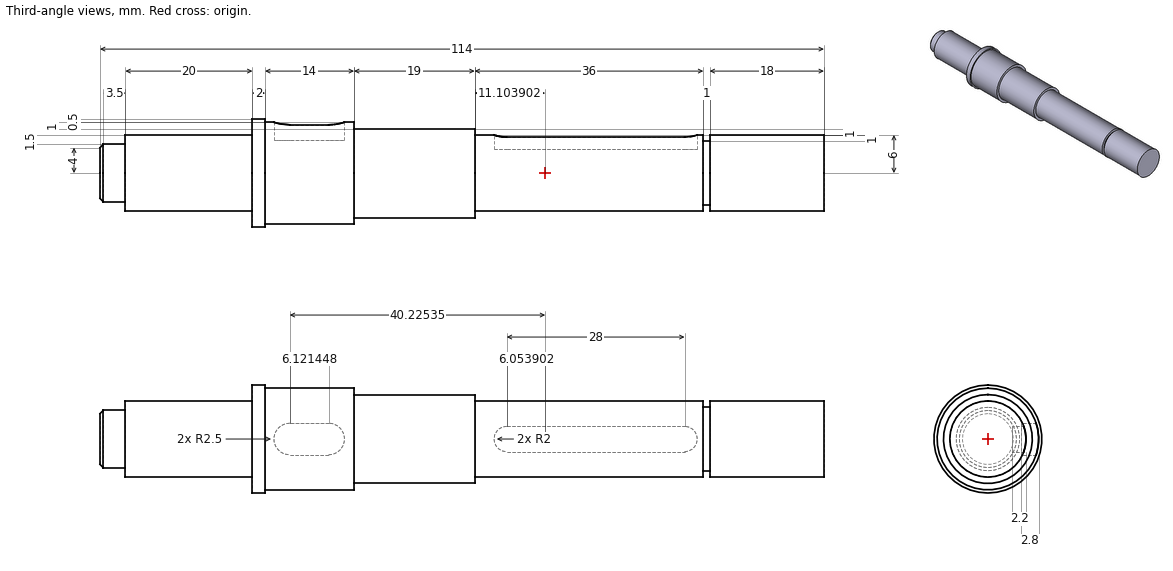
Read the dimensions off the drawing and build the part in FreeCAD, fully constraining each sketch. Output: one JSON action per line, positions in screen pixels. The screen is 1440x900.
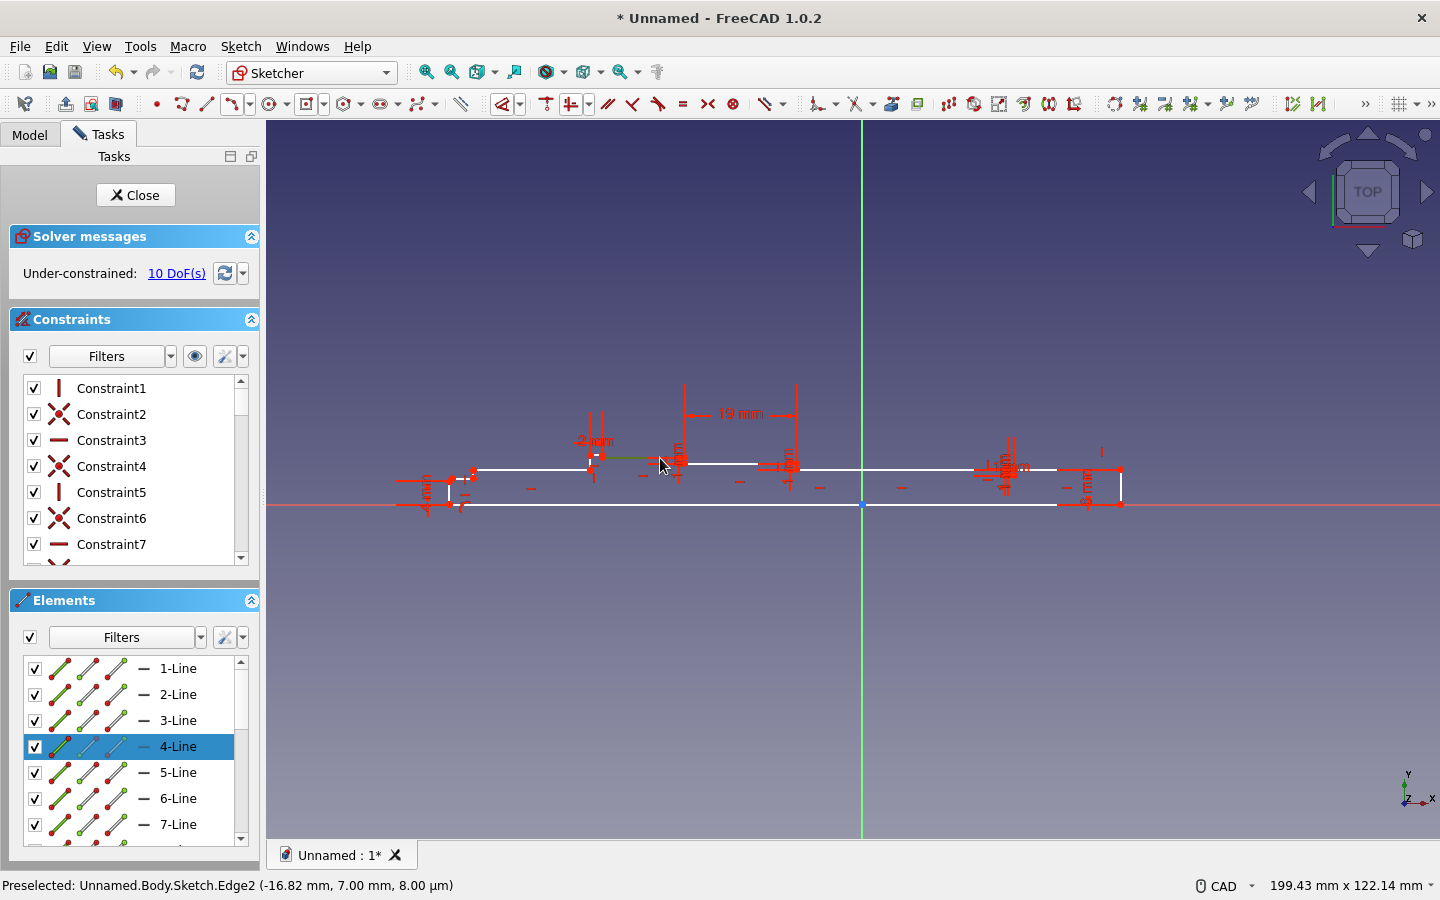
{"action": "key", "text": "l"}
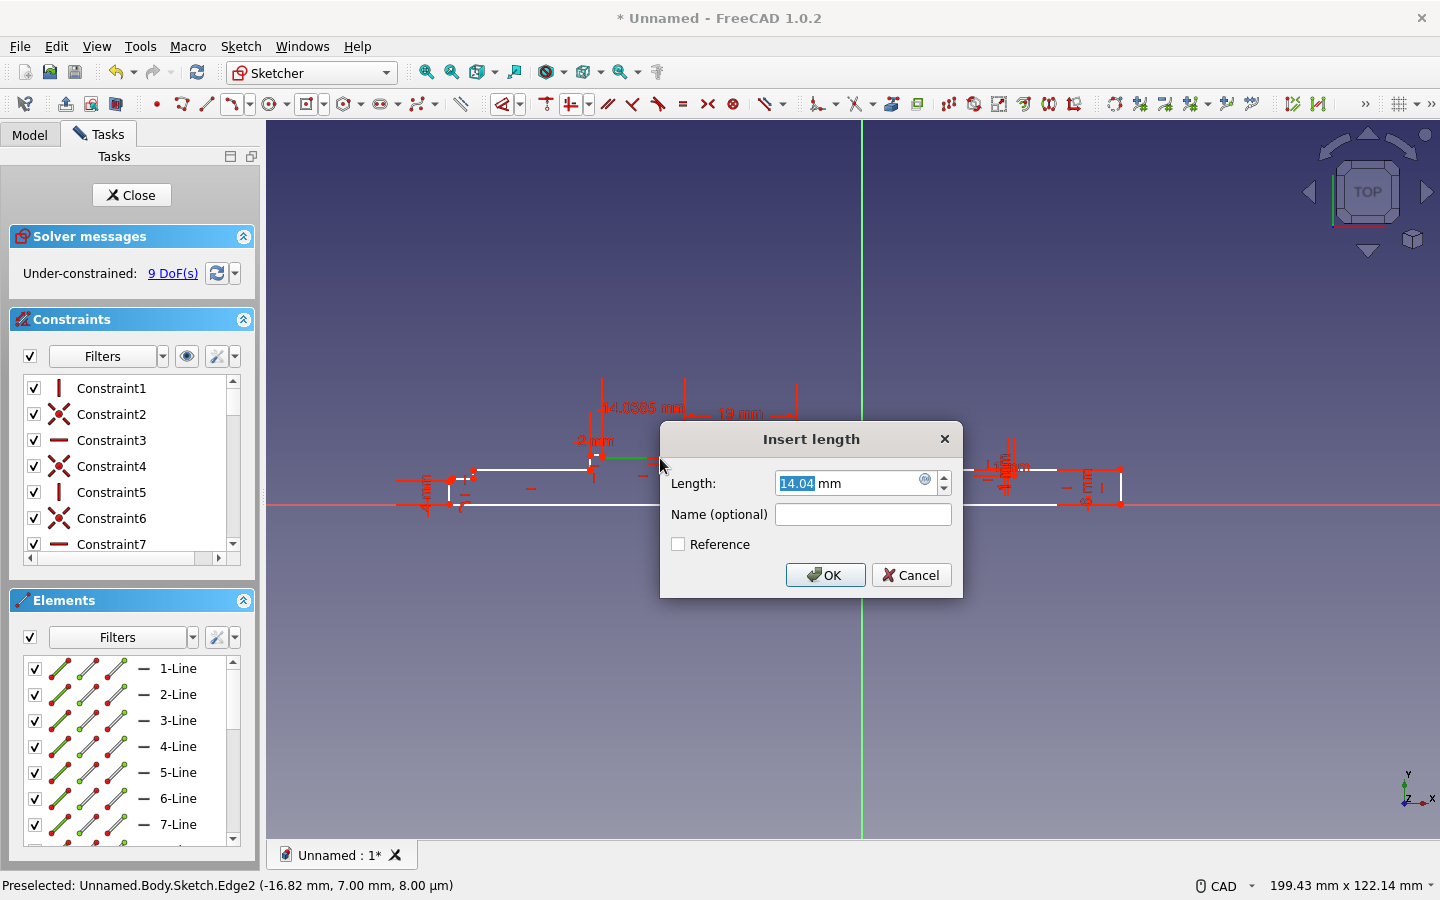
{"action": "type", "text": "14"}
{"action": "key", "text": "Return"}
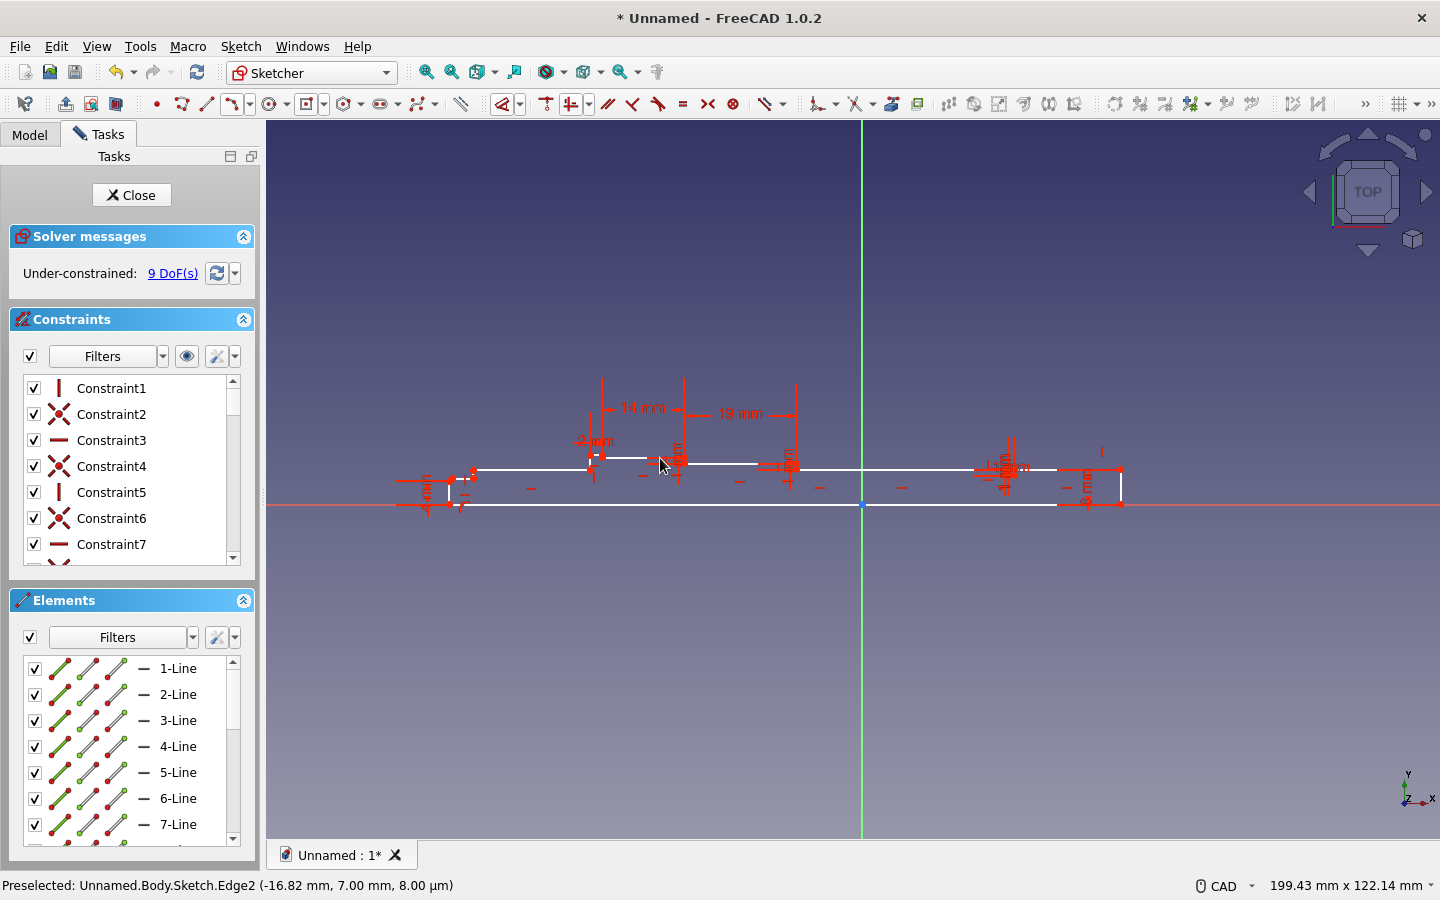
{"action": "left_click", "coordinate": [555, 470]}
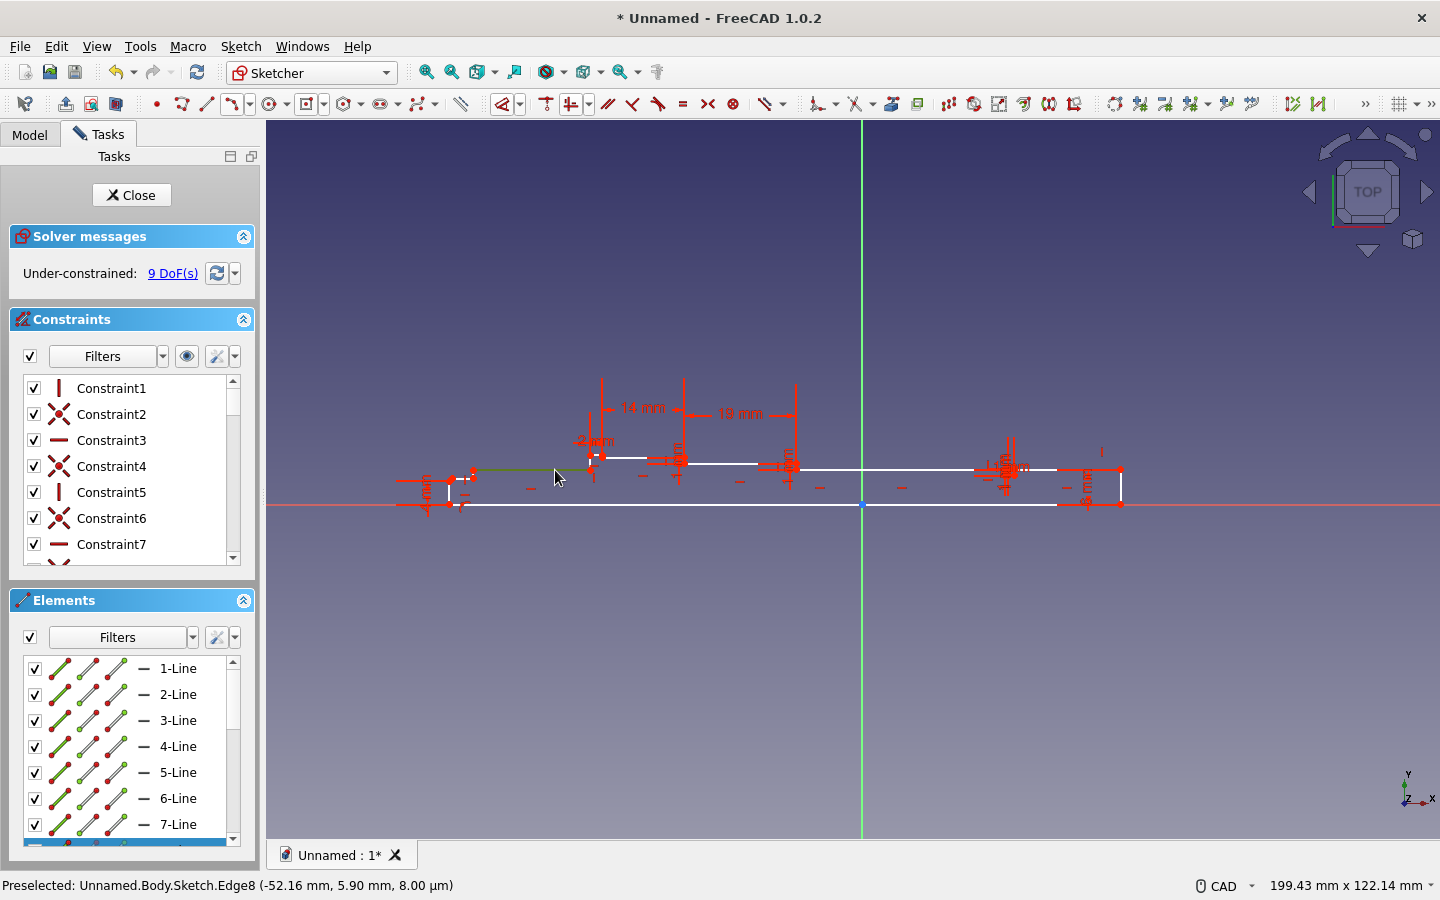
{"action": "key", "text": "l"}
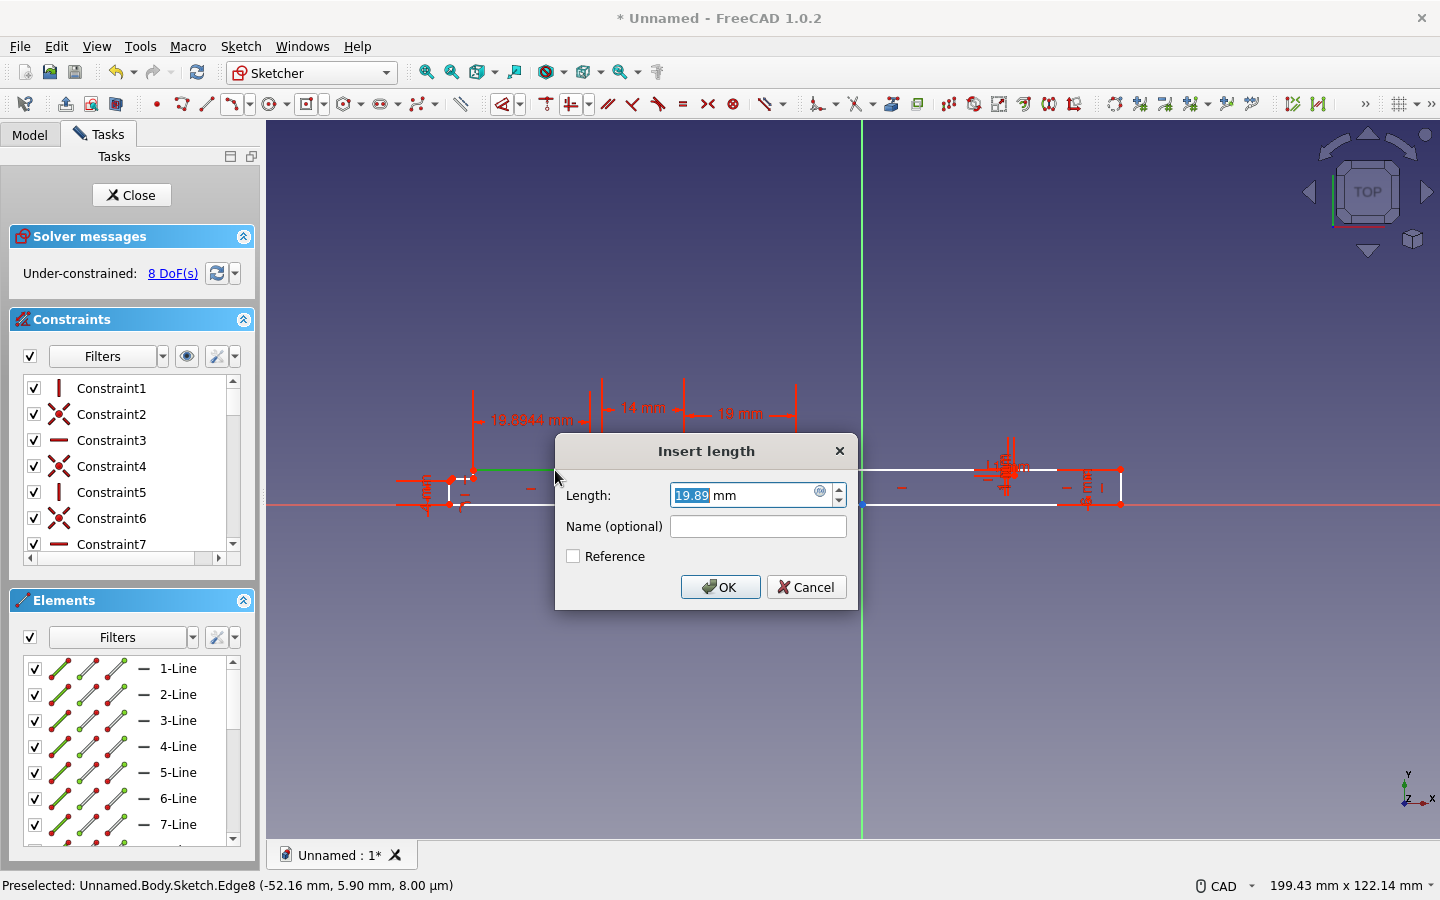
{"action": "type", "text": "20"}
{"action": "key", "text": "Return"}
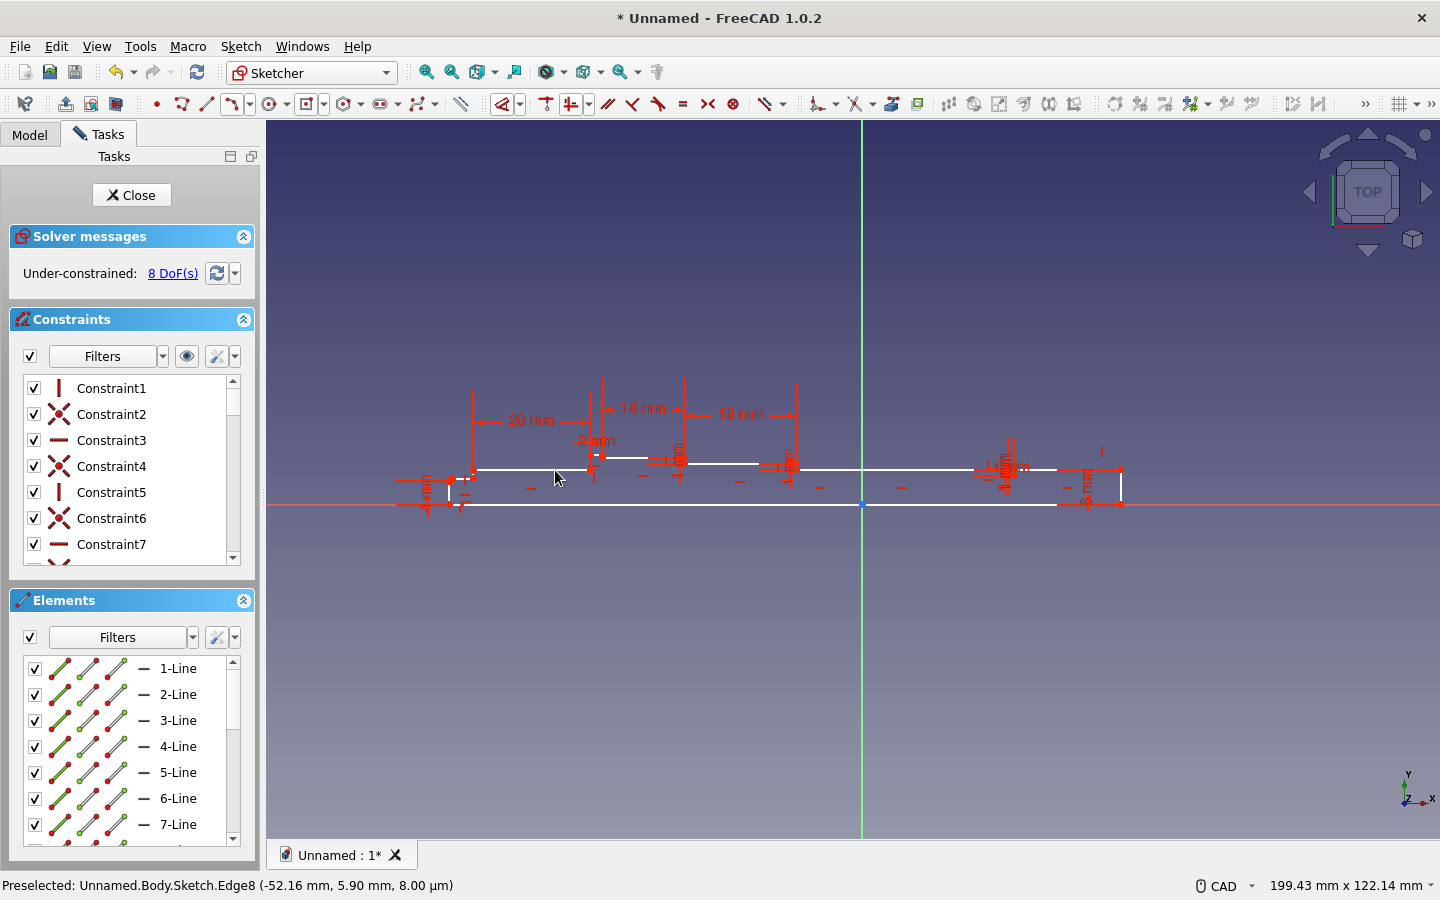
{"action": "left_click", "coordinate": [1046, 470]}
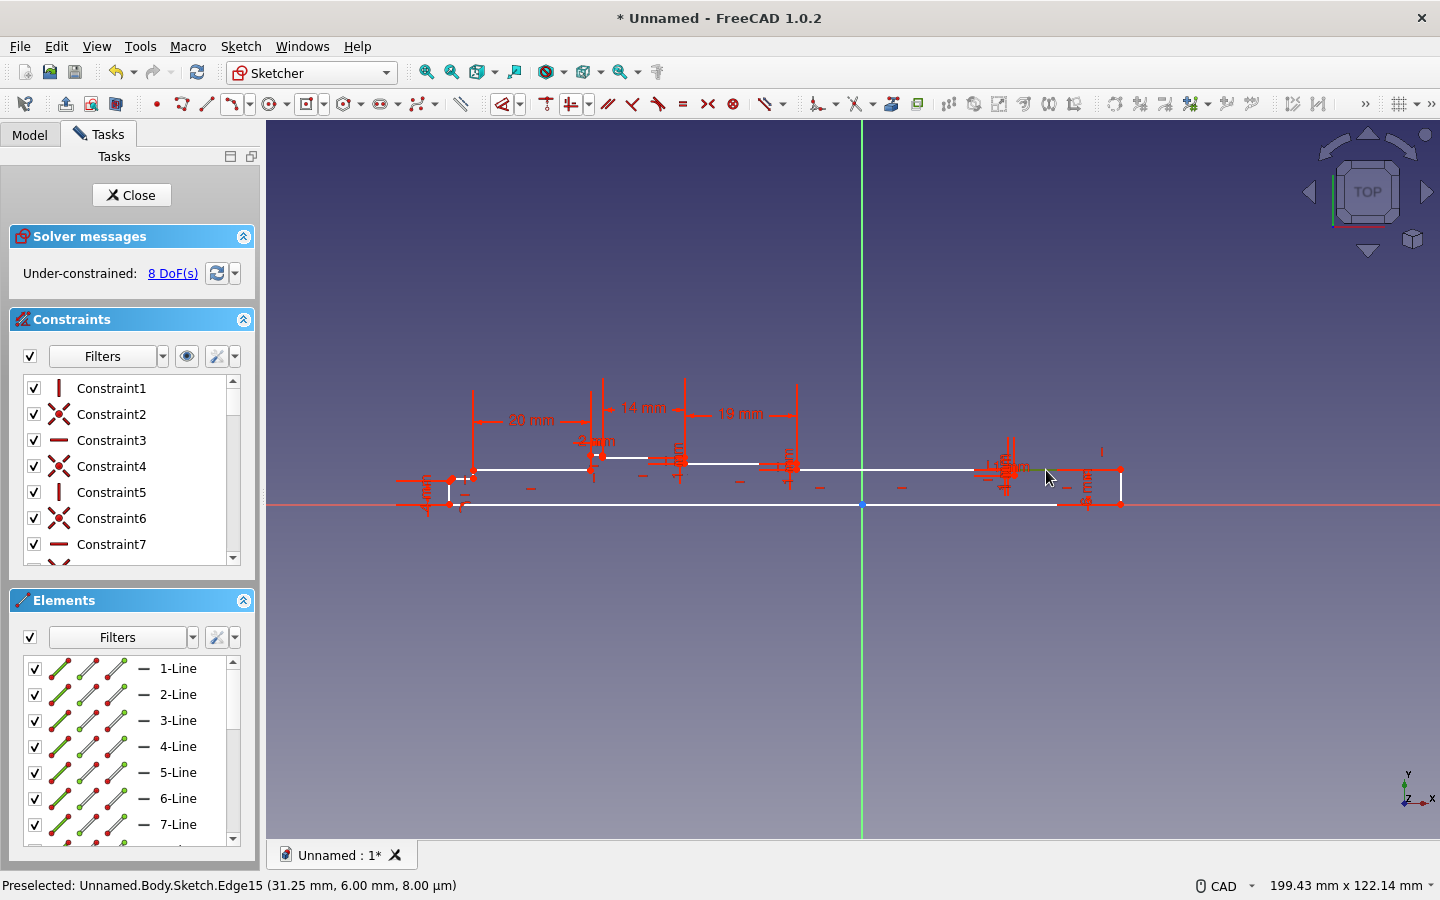
{"action": "left_click", "coordinate": [520, 104]}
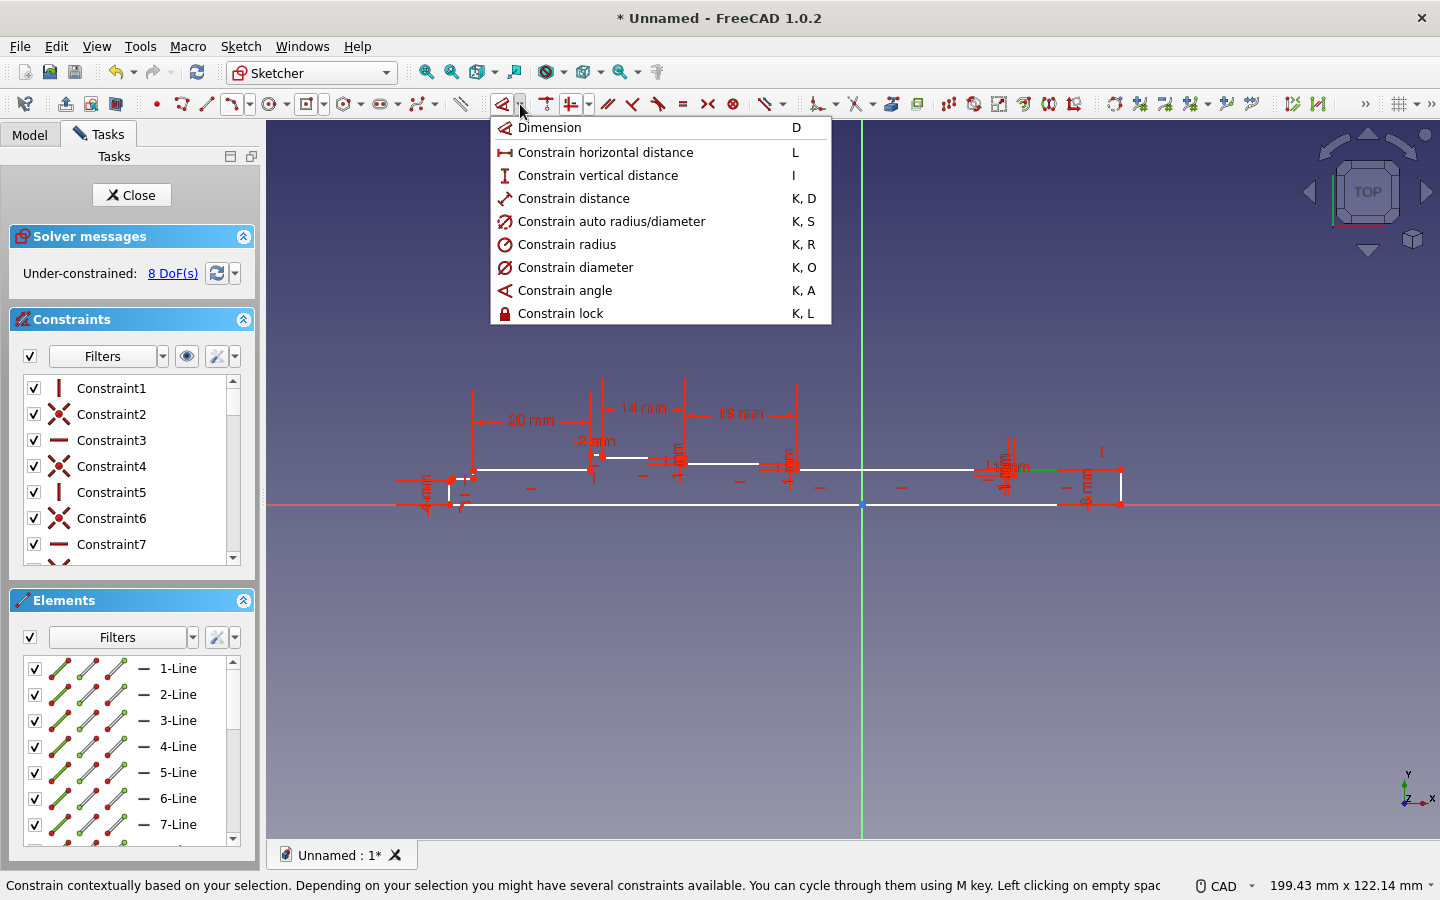
{"action": "left_click", "coordinate": [661, 152]}